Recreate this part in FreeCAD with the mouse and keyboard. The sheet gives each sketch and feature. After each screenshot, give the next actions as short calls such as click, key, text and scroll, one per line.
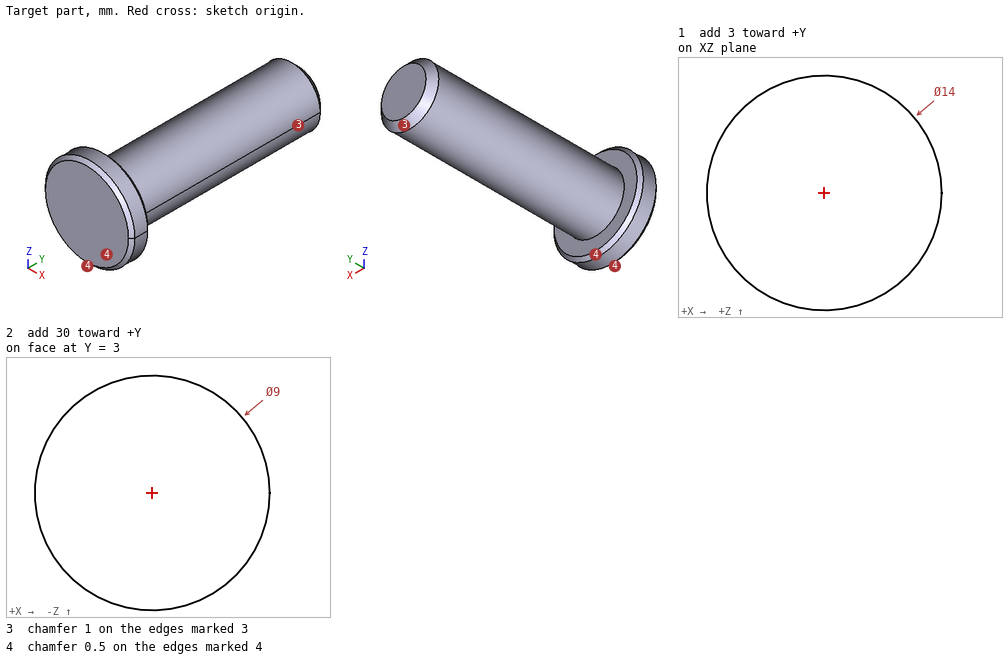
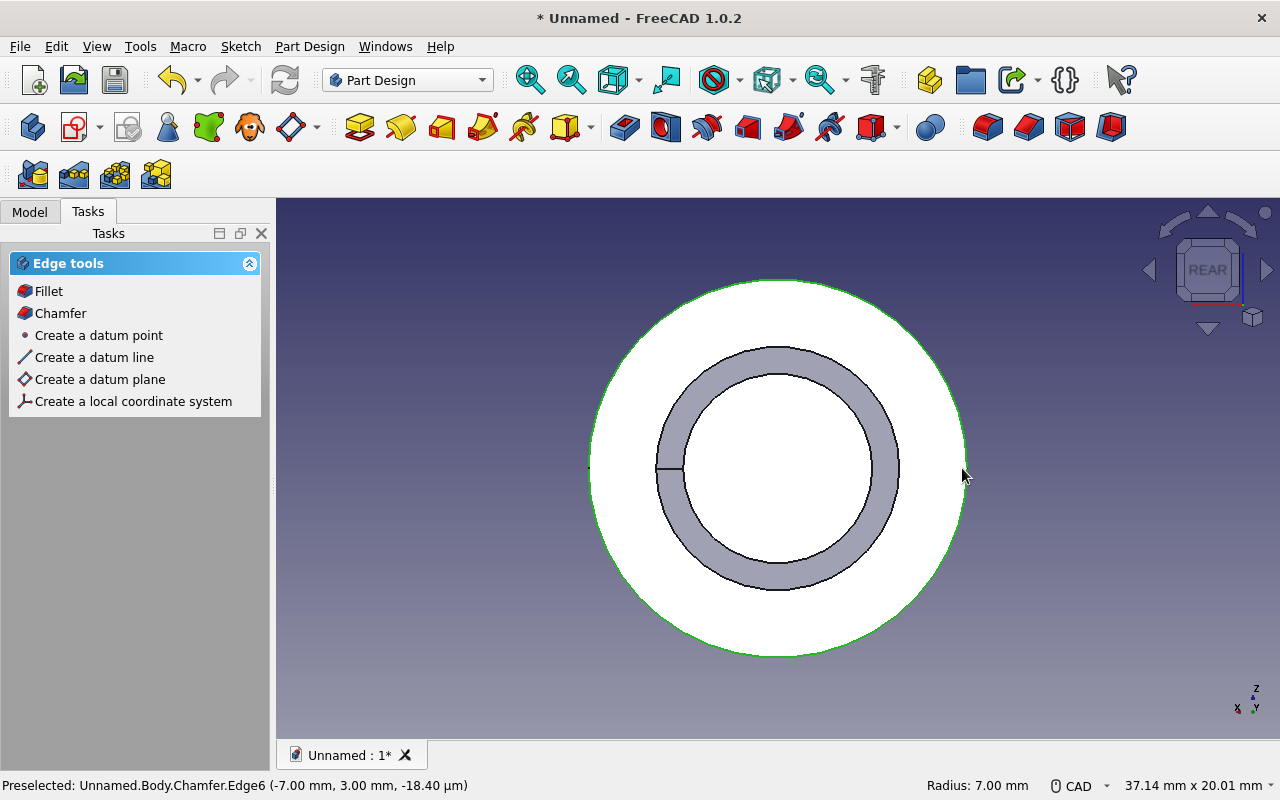
key(0)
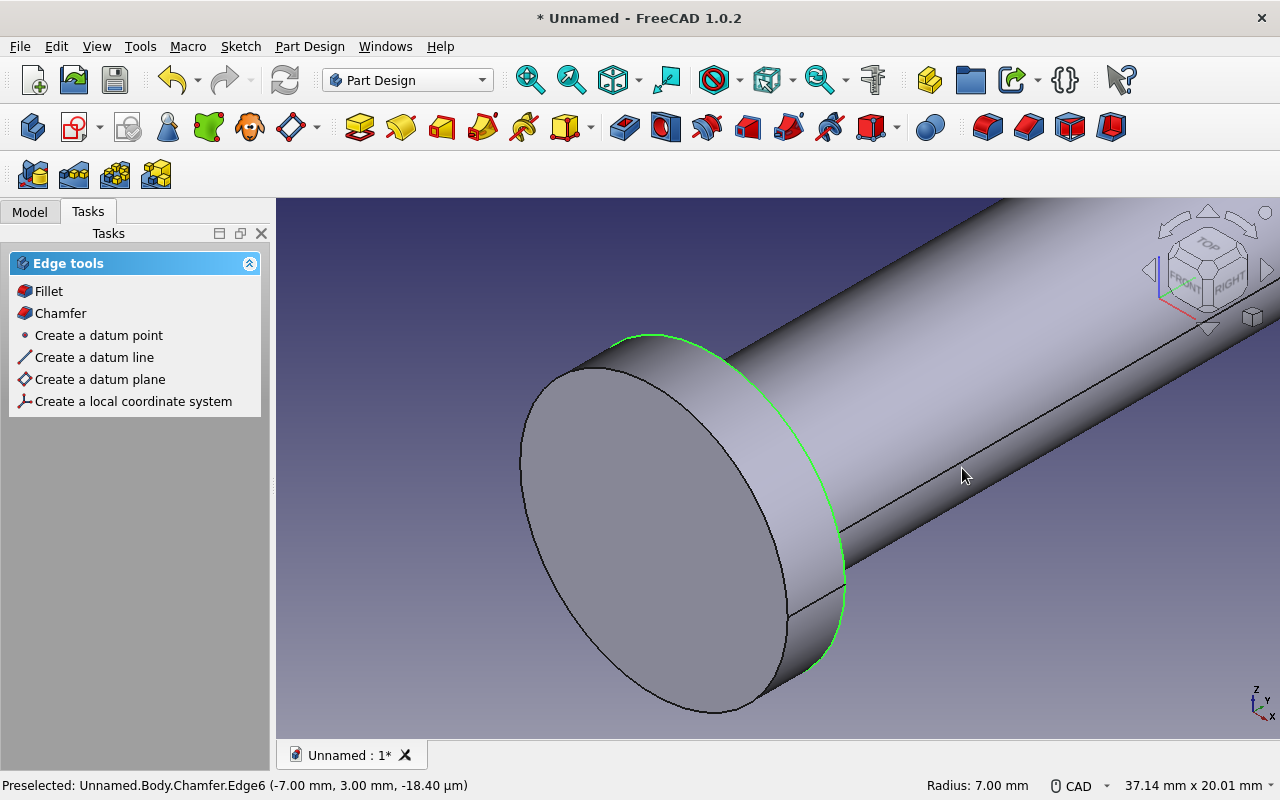
click(531, 80)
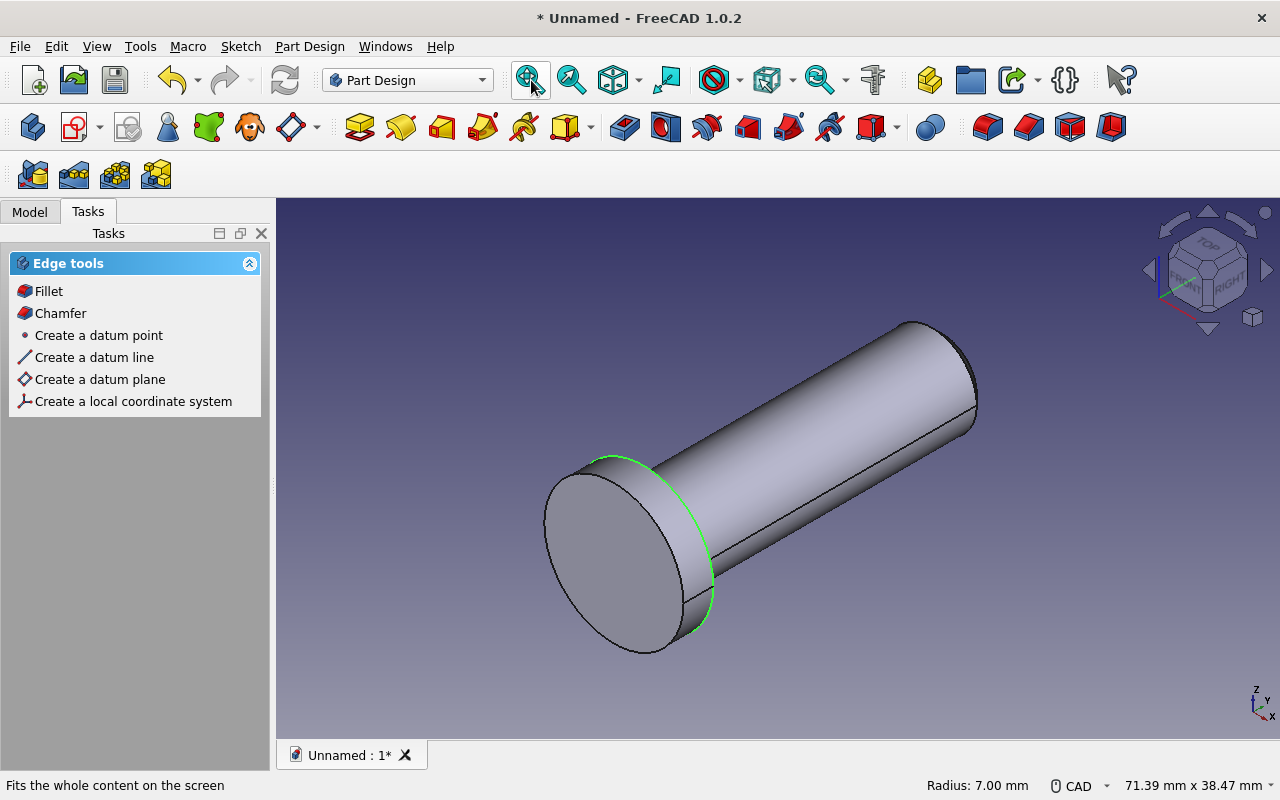
click(592, 473, ctrl)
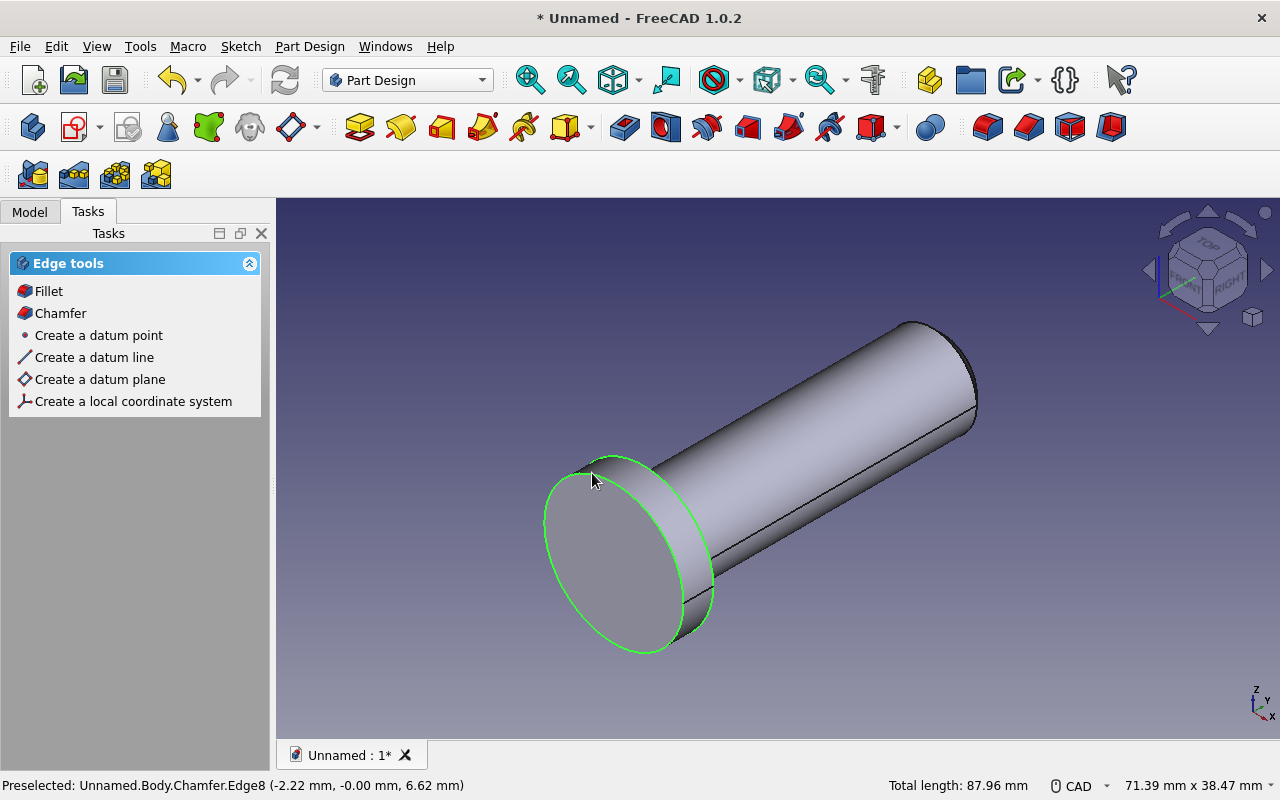
click(1029, 128)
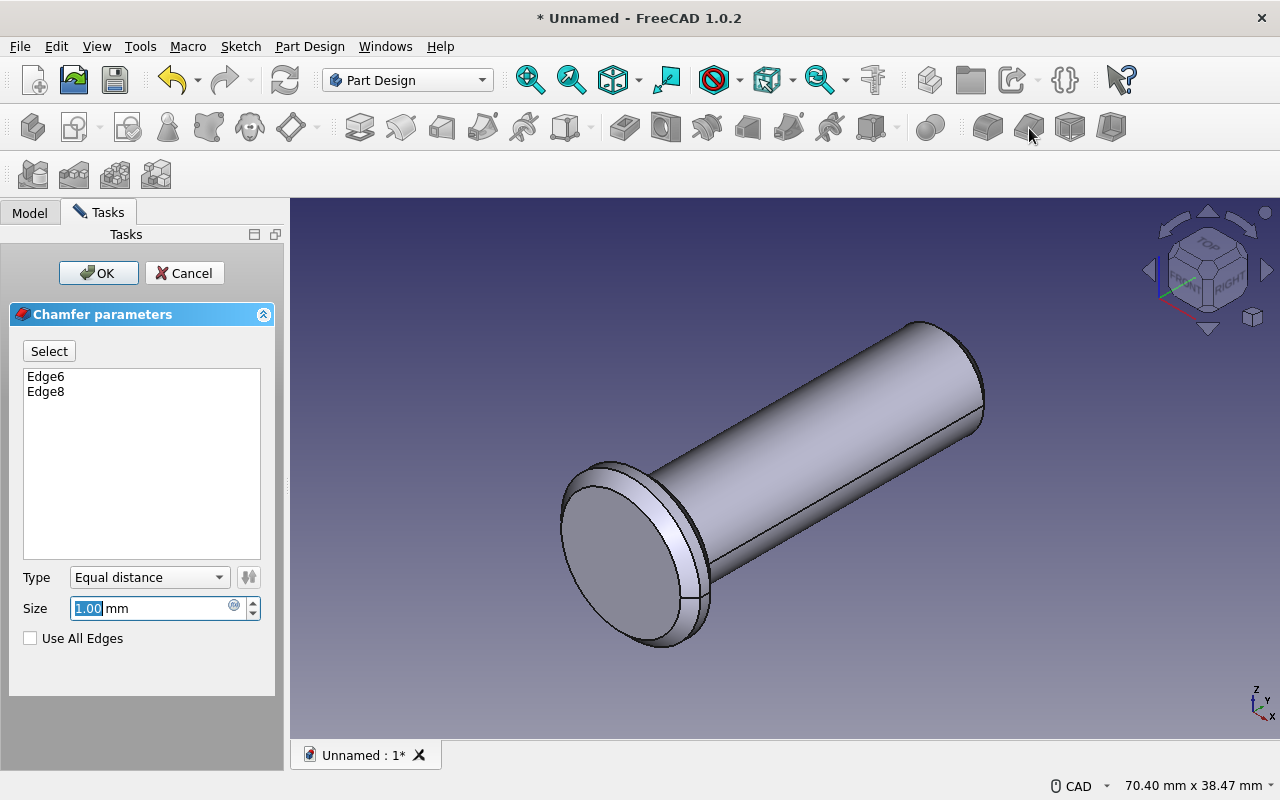
text(0.5)
key(Tab)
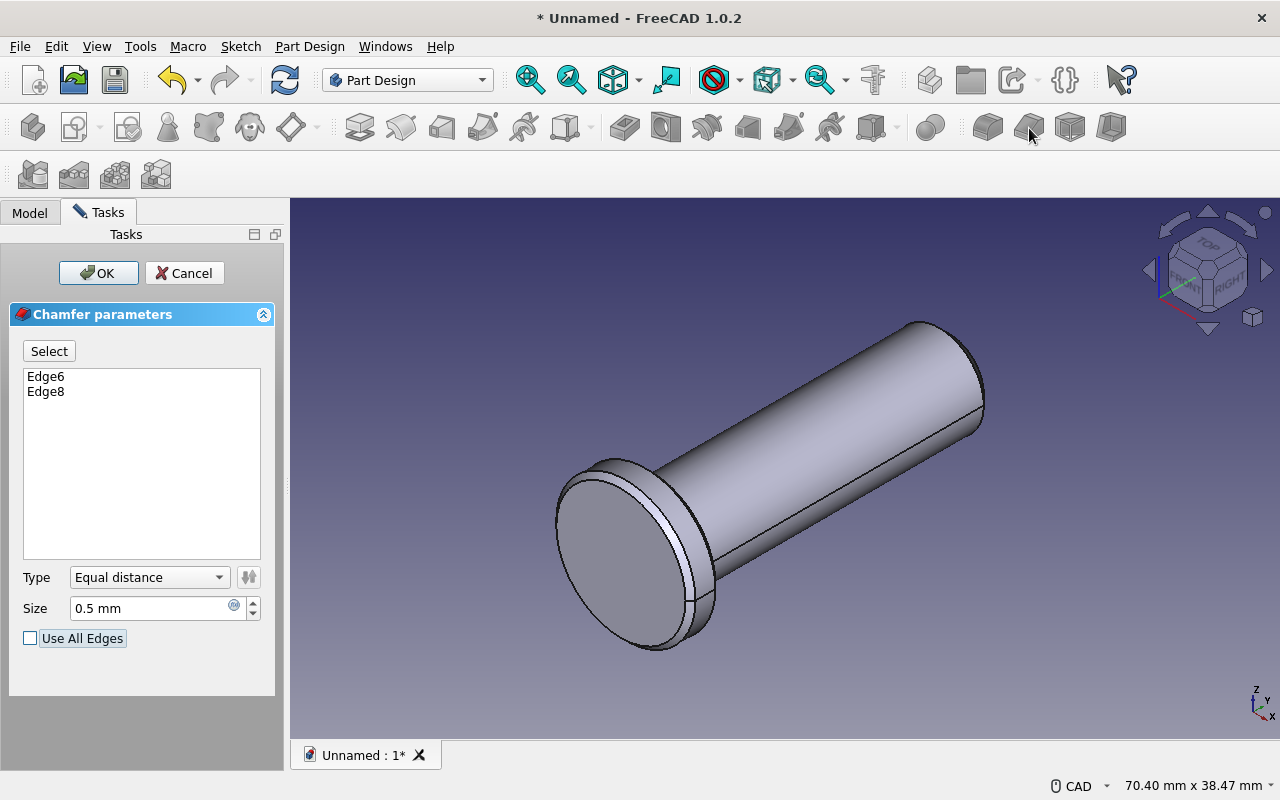
click(99, 273)